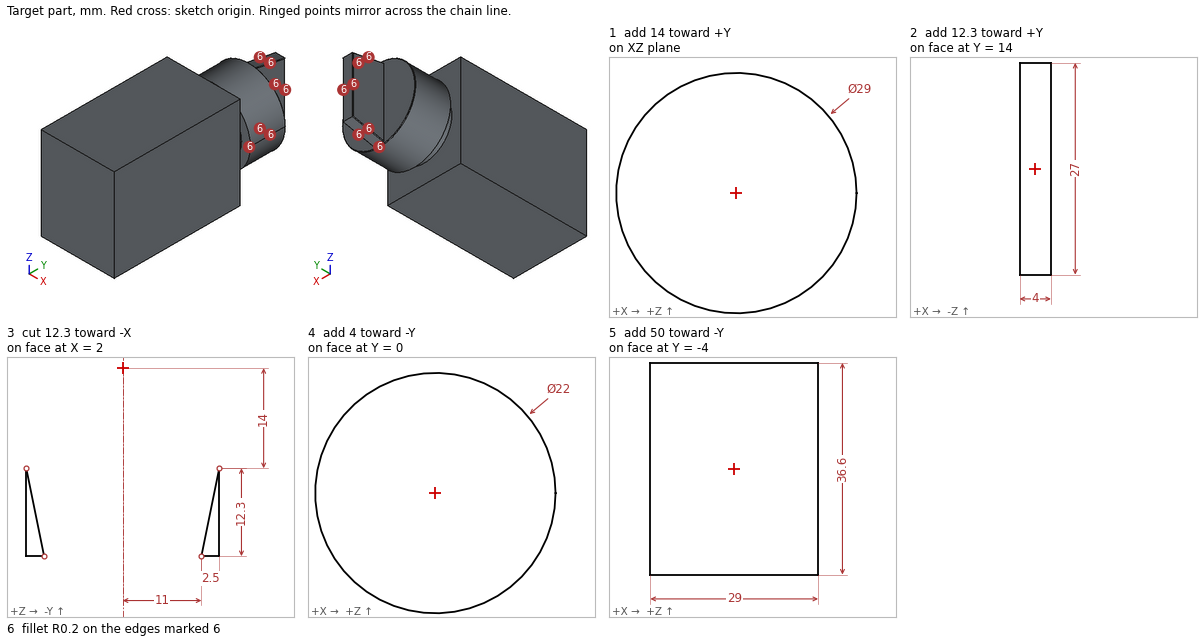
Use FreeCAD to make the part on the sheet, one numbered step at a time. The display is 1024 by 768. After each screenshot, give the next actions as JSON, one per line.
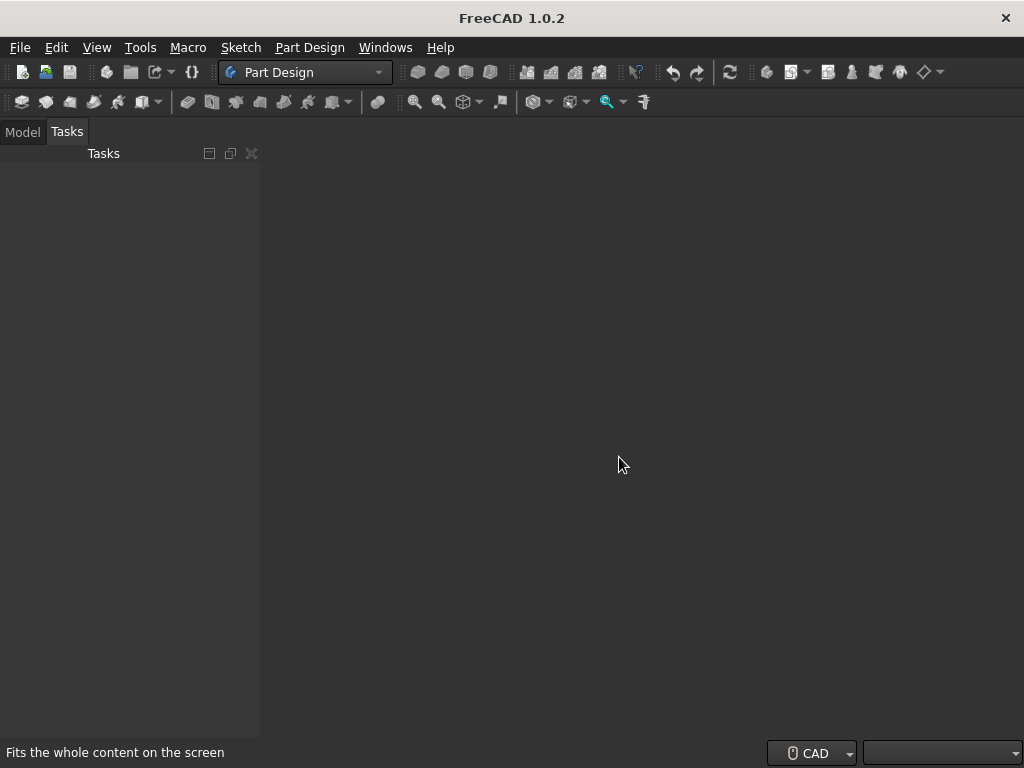
{"action": "key", "text": "ctrl+n"}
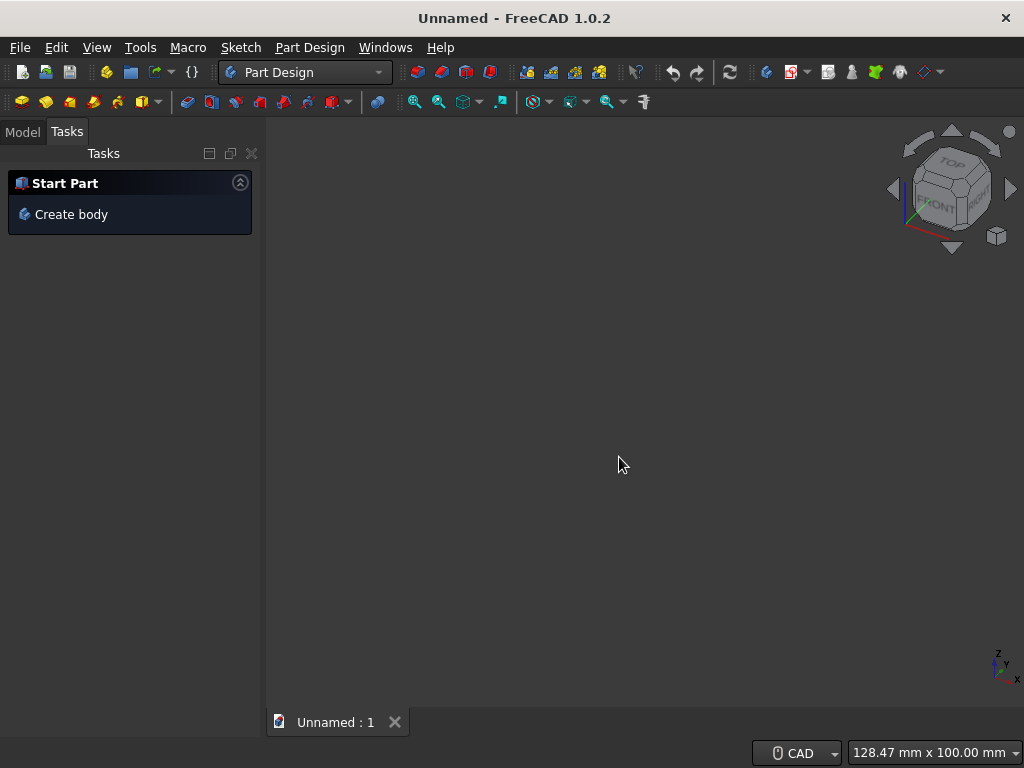
{"action": "left_click", "coordinate": [792, 72]}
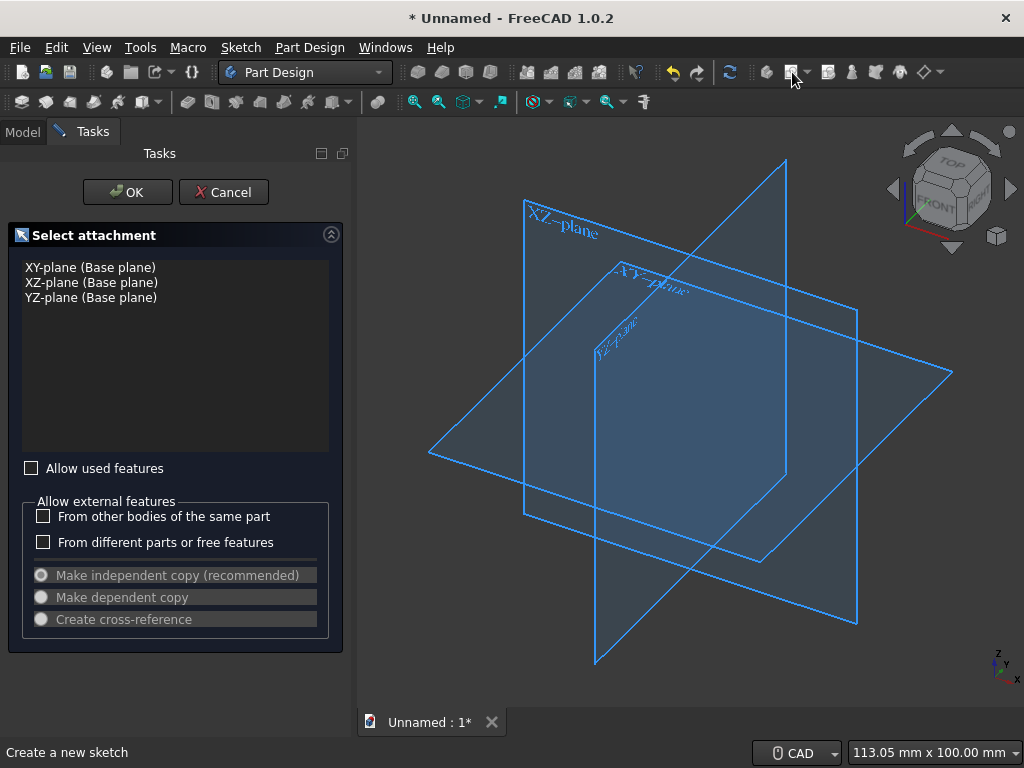
{"action": "left_click", "coordinate": [82, 282]}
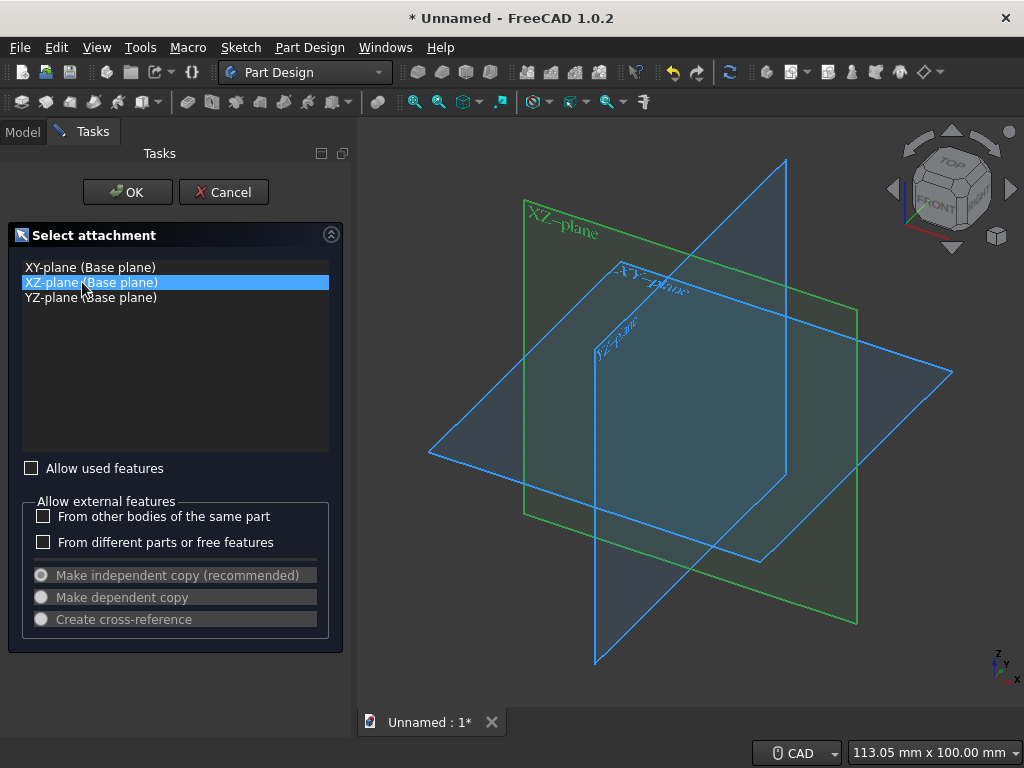
{"action": "left_click", "coordinate": [128, 192]}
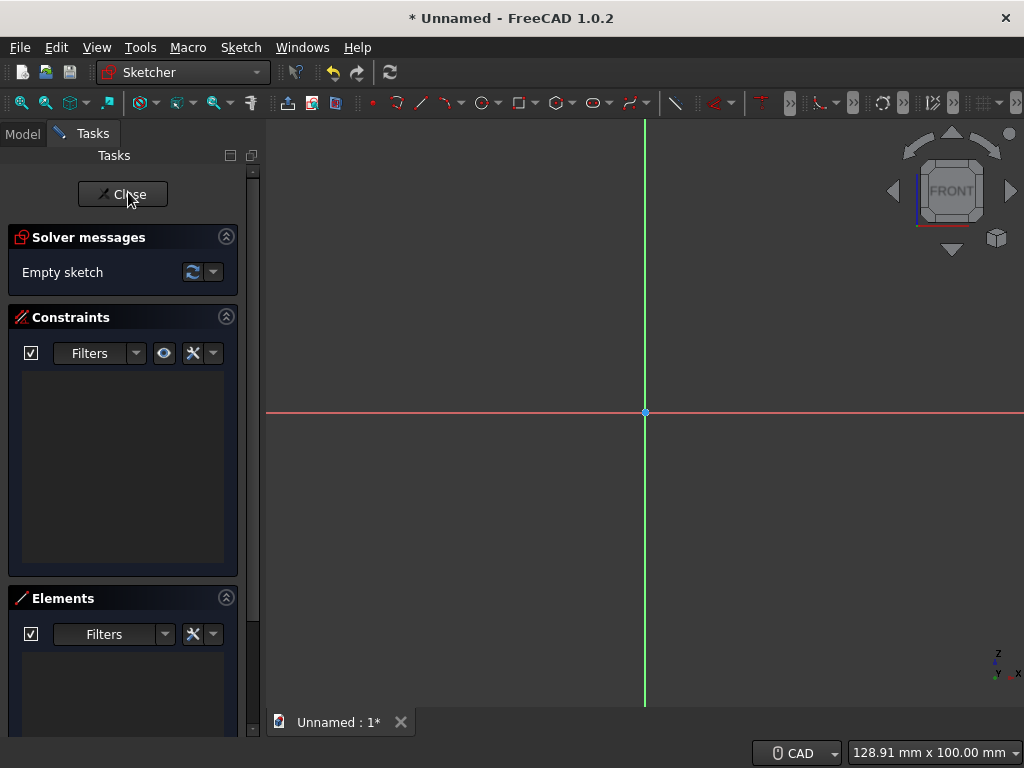
{"action": "scroll", "coordinate": [701, 413], "scroll_direction": "up", "scroll_amount": 4}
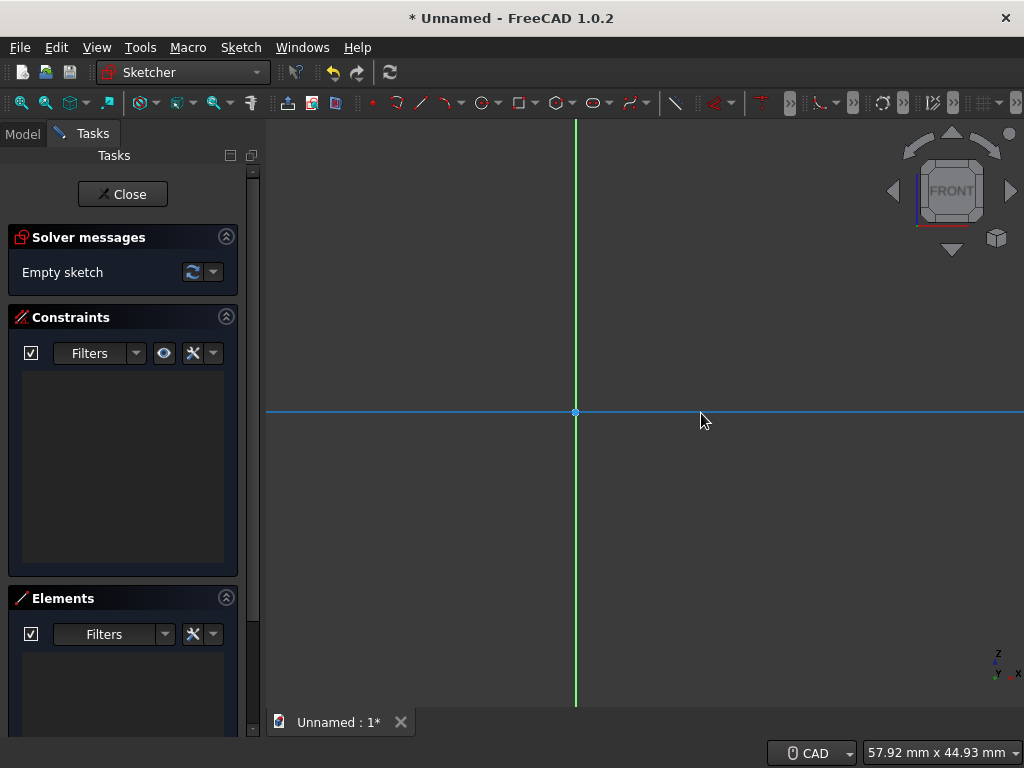
{"action": "key", "text": "g c"}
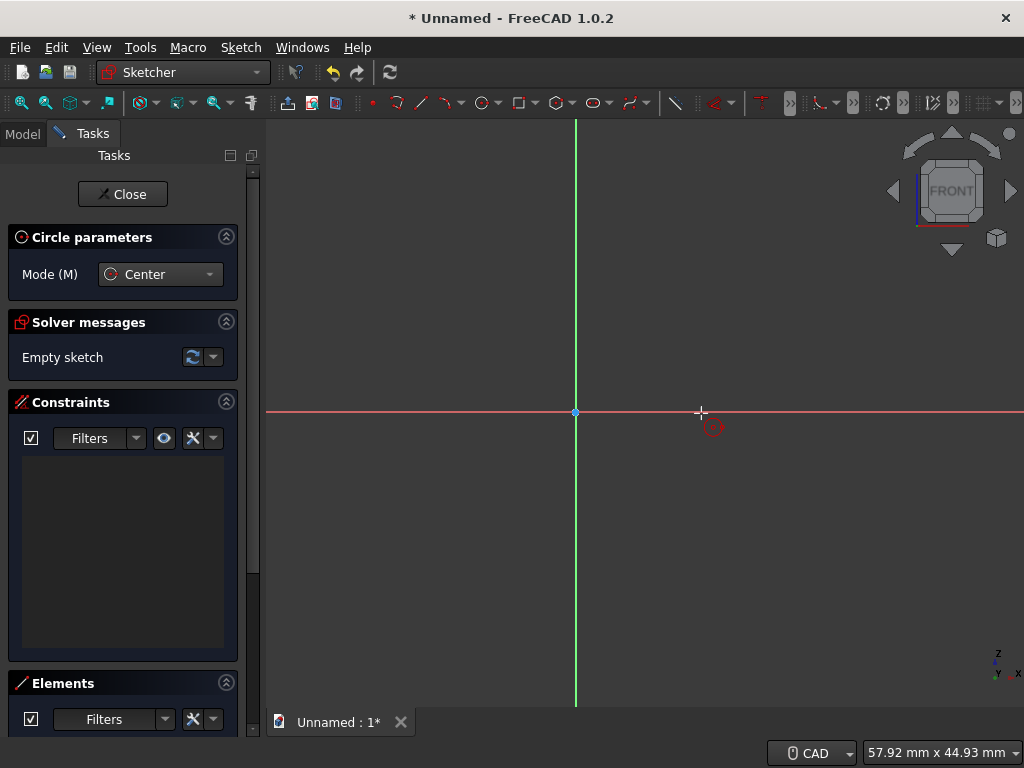
{"action": "left_click", "coordinate": [576, 412]}
{"action": "mouse_move", "coordinate": [710, 278]}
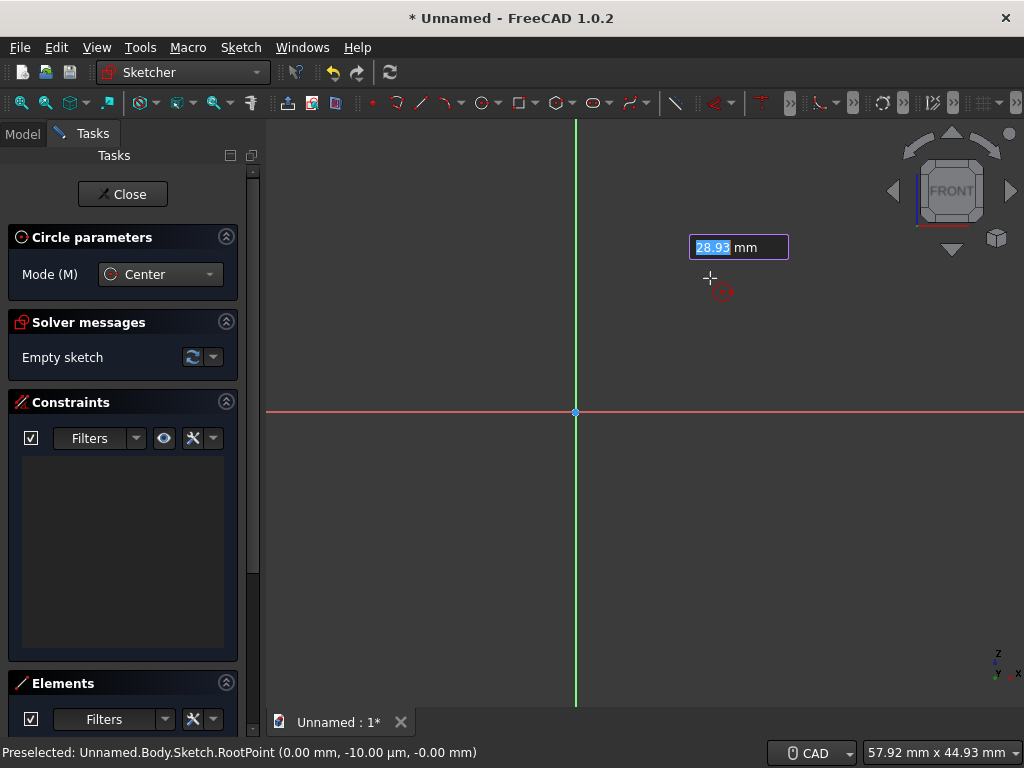
{"action": "type", "text": "29"}
{"action": "key", "text": "Return"}
{"action": "key", "text": "Escape"}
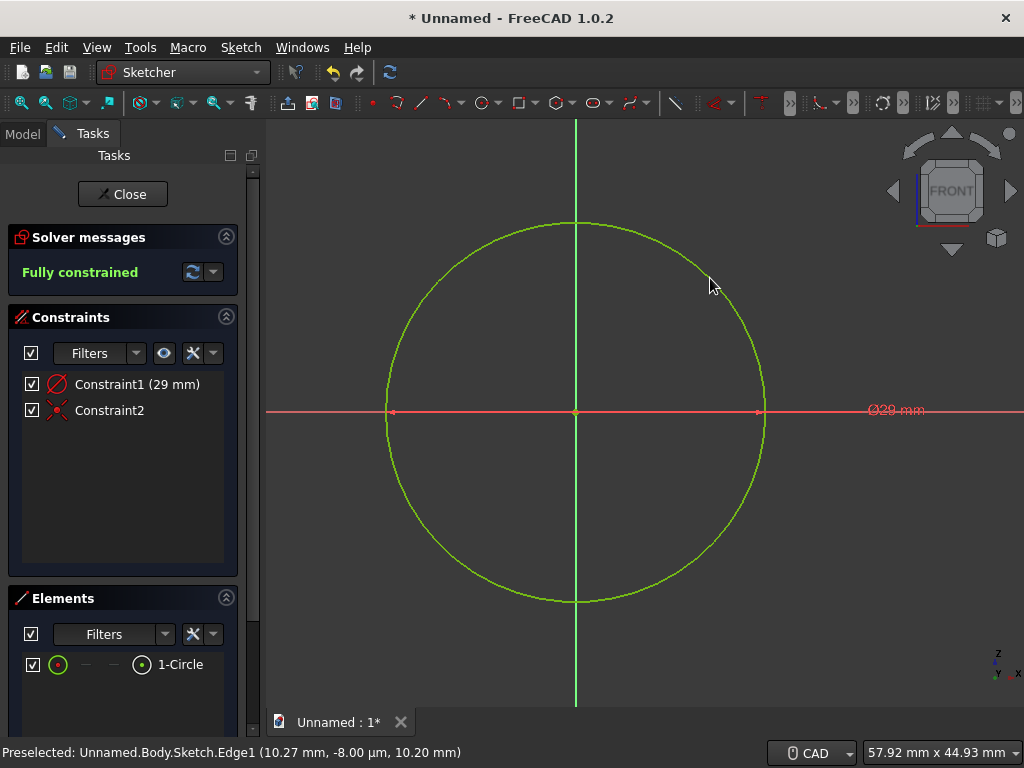
{"action": "left_click", "coordinate": [123, 194]}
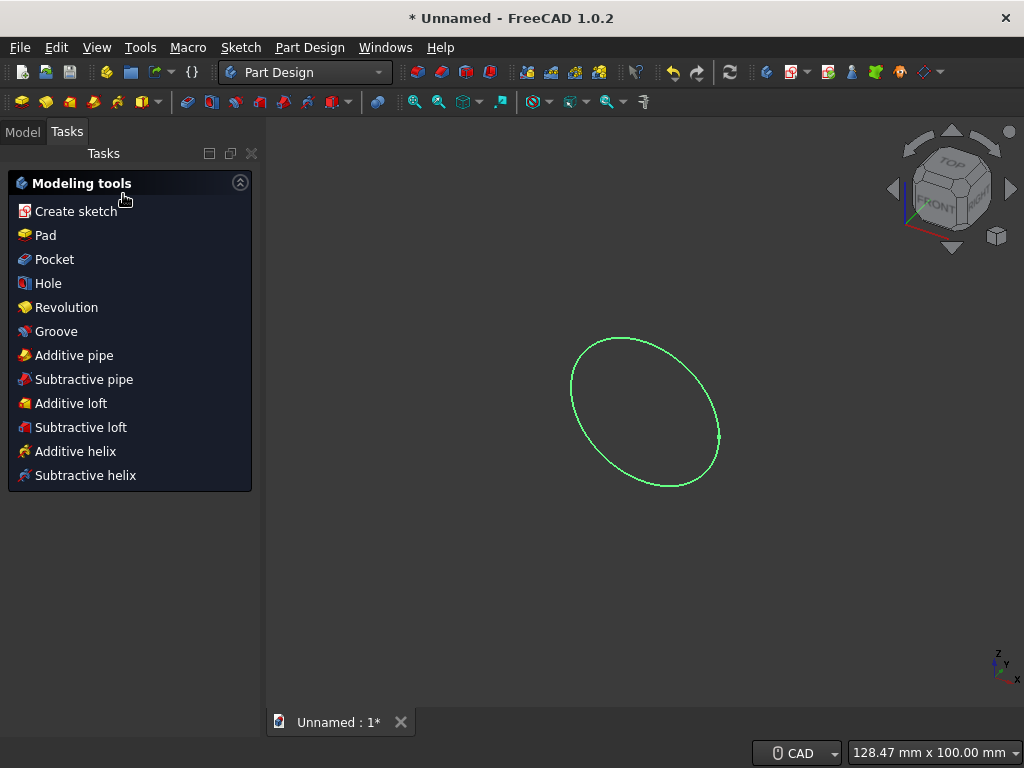
{"action": "left_click", "coordinate": [22, 102]}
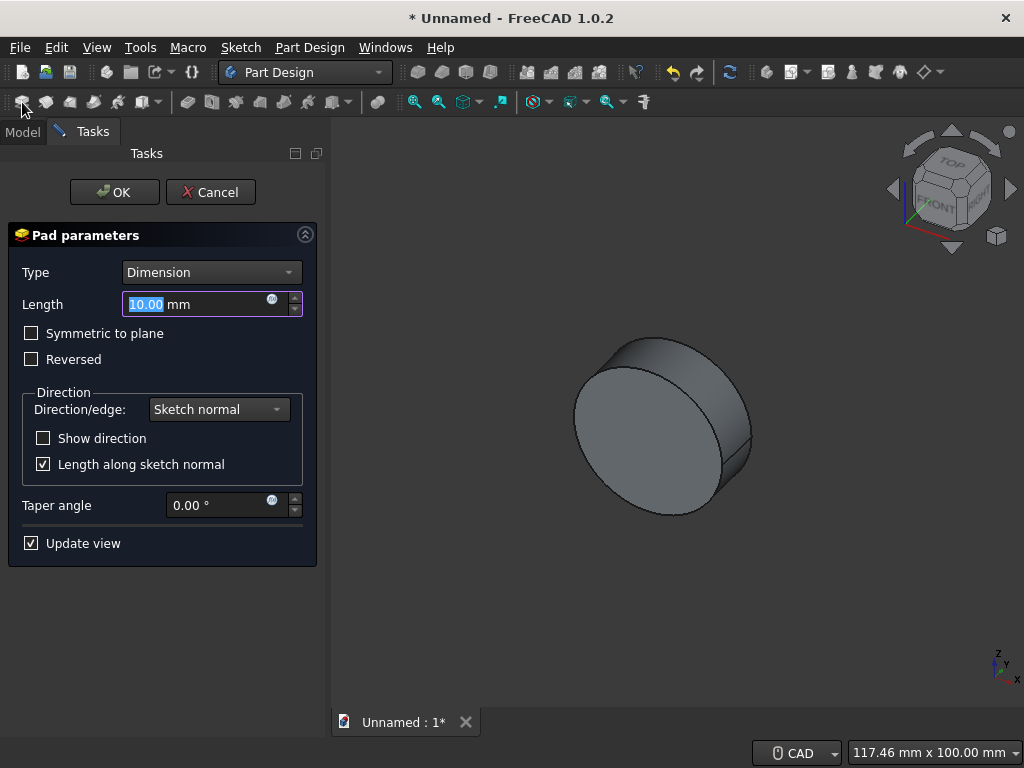
{"action": "type", "text": "14"}
{"action": "key", "text": "Tab"}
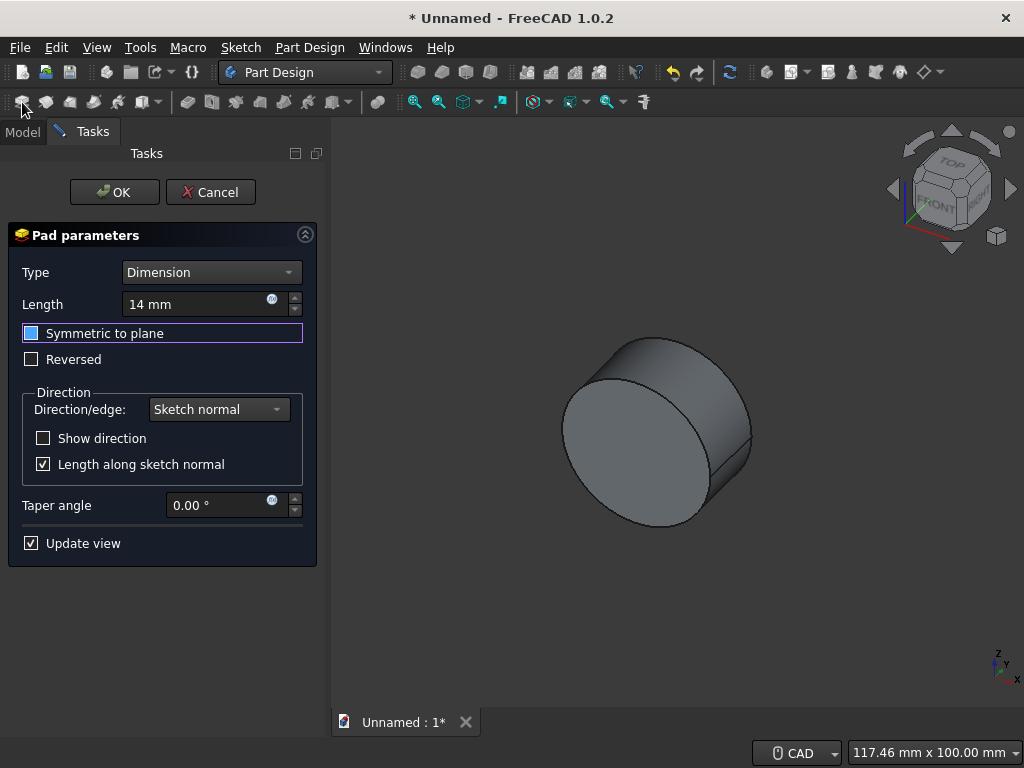
{"action": "left_click", "coordinate": [30, 359]}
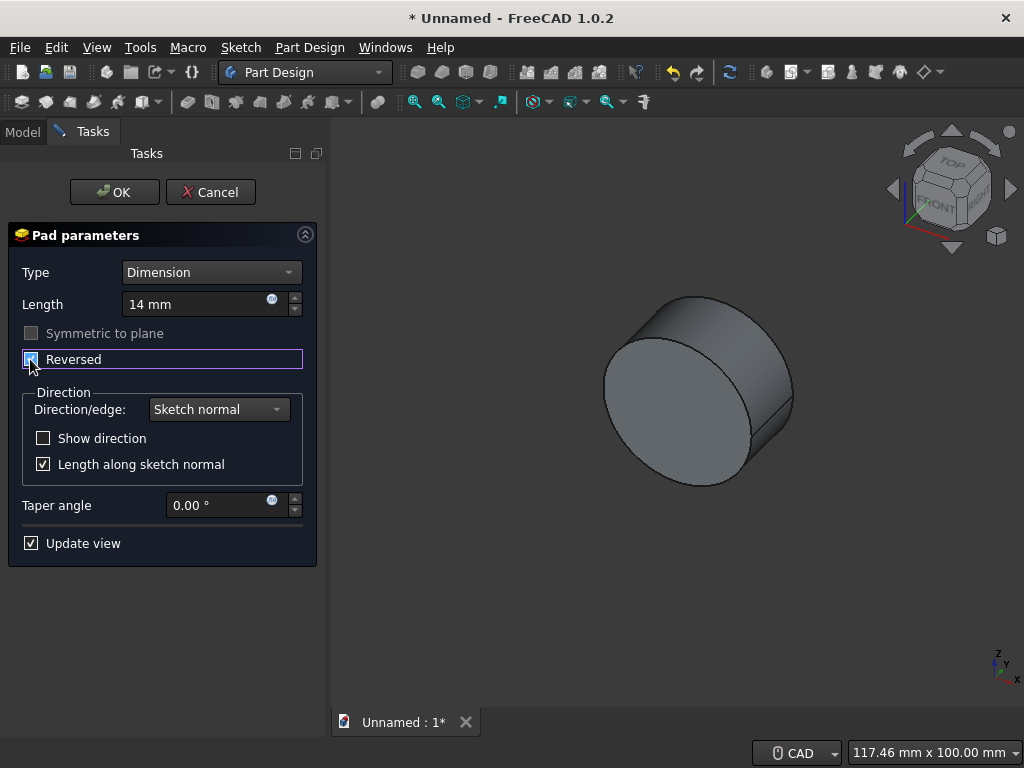
{"action": "left_click", "coordinate": [115, 192]}